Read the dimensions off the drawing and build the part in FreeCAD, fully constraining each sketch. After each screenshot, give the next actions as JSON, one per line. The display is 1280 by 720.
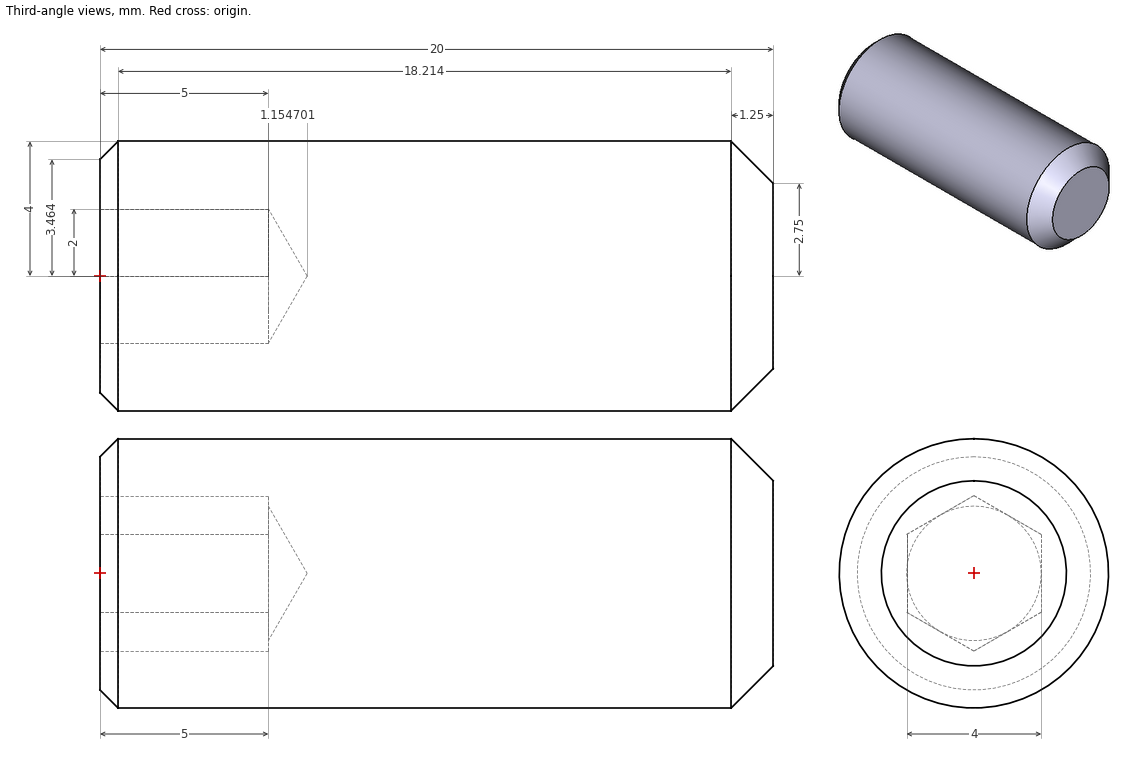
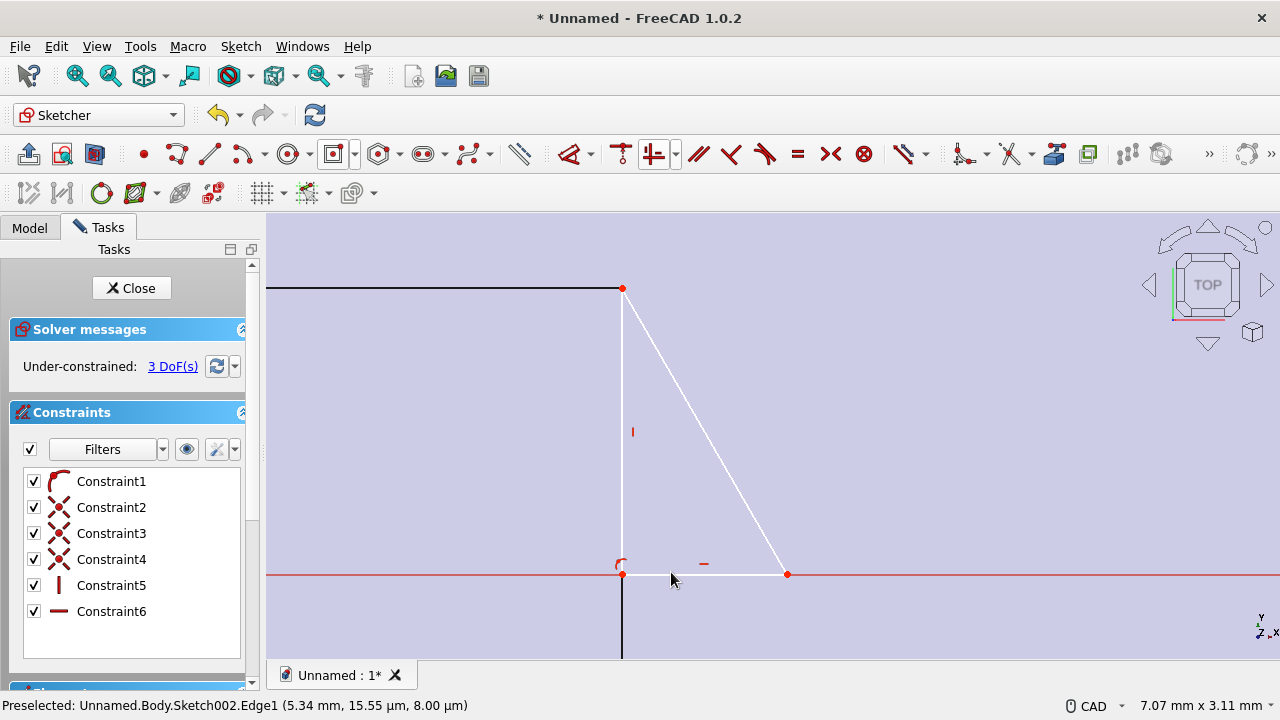
{"action": "left_click", "coordinate": [568, 154]}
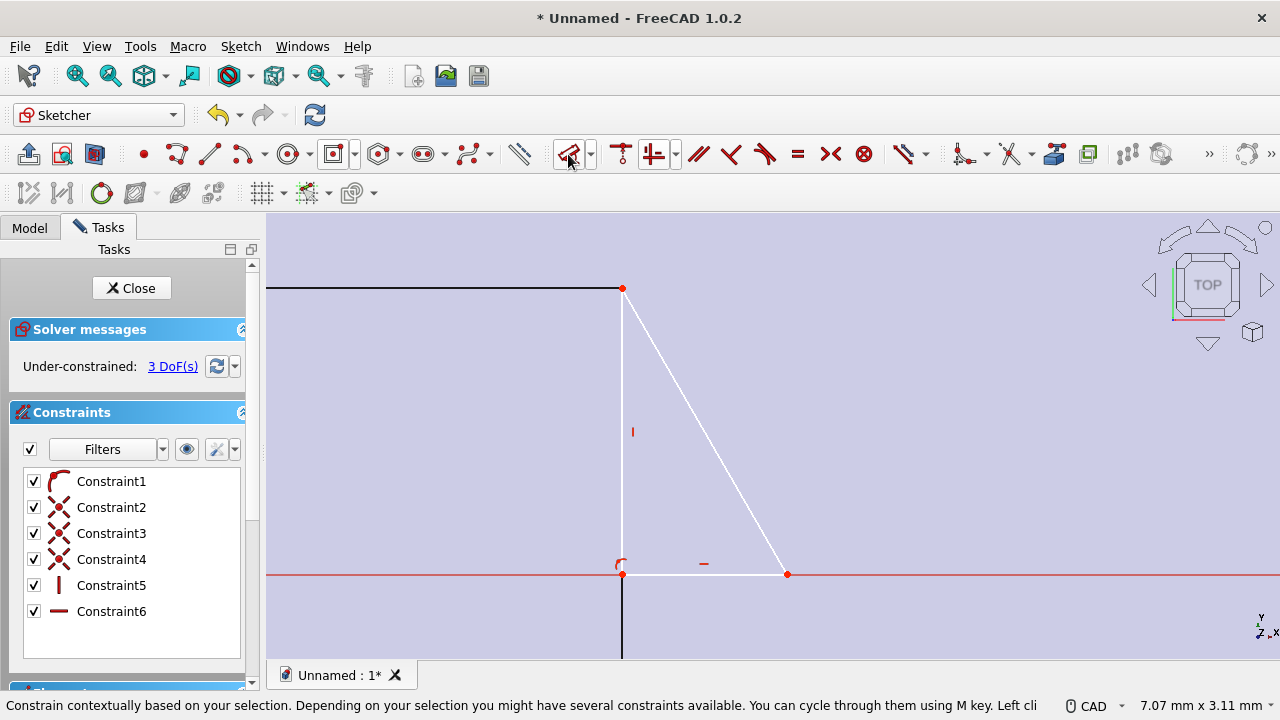
{"action": "left_click", "coordinate": [622, 375]}
{"action": "left_click", "coordinate": [588, 432]}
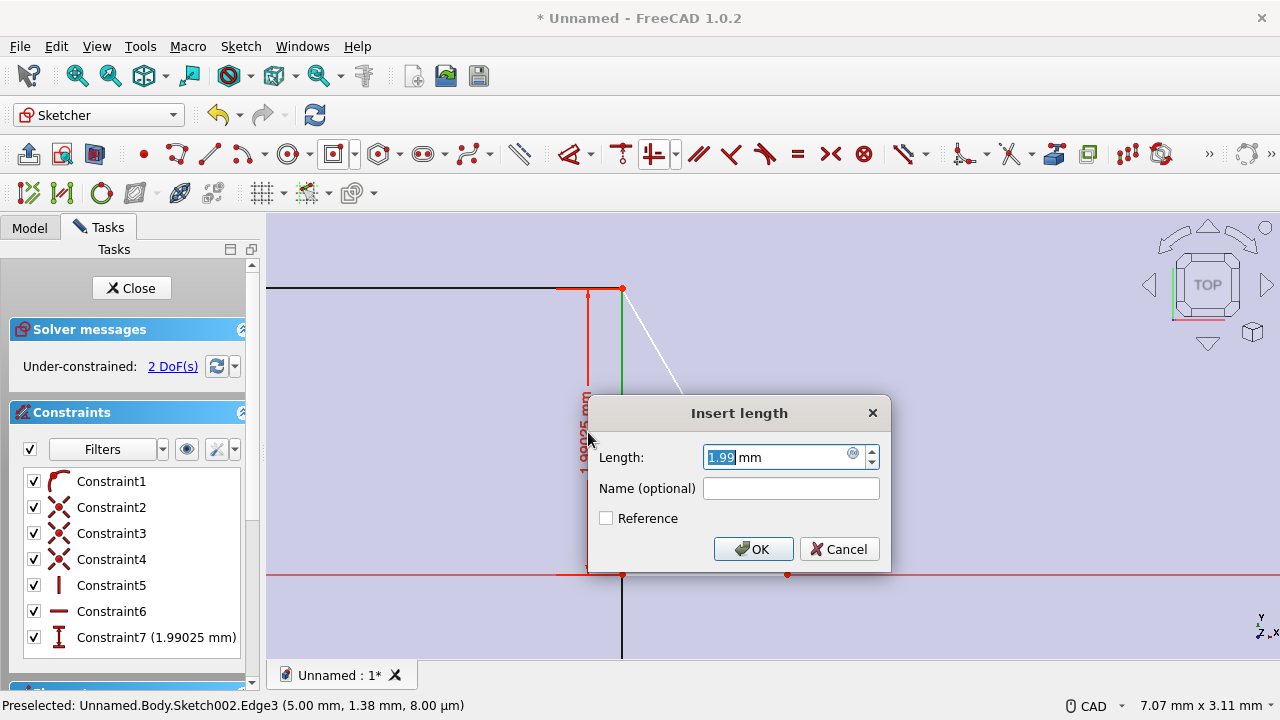
{"action": "type", "text": "2"}
{"action": "key", "text": "Return"}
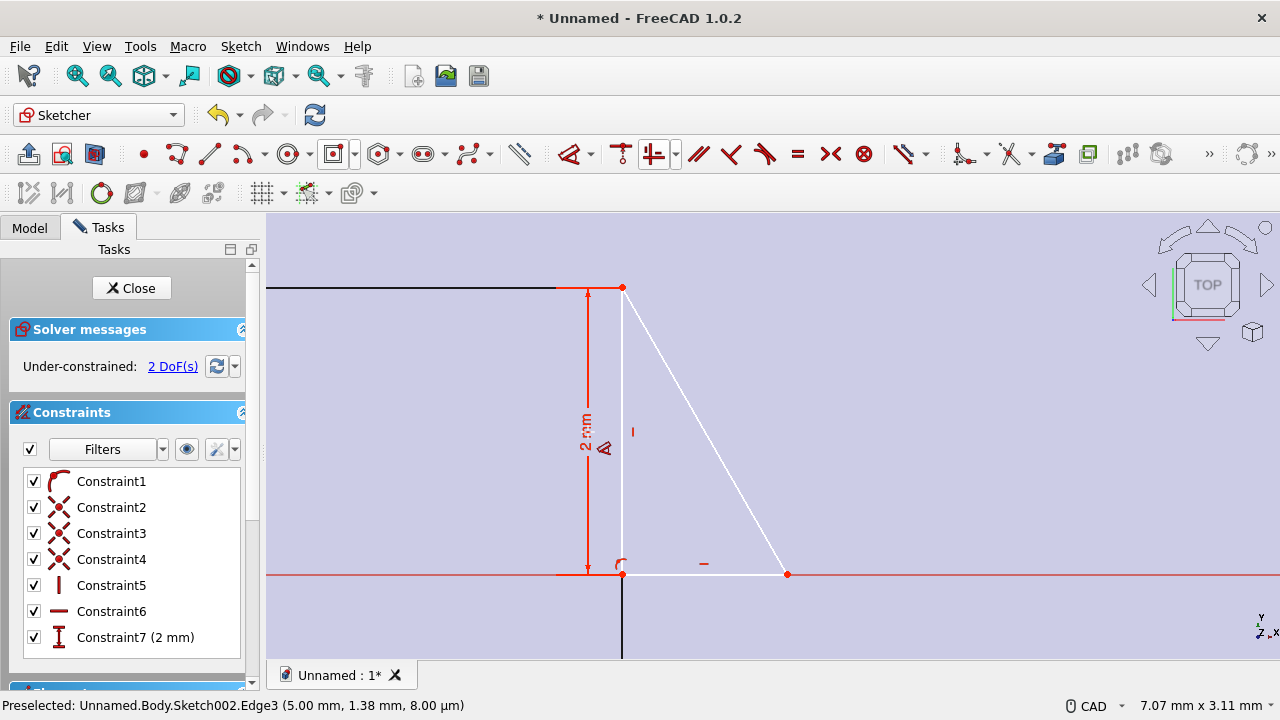
{"action": "left_click", "coordinate": [622, 575]}
{"action": "left_click", "coordinate": [458, 609]}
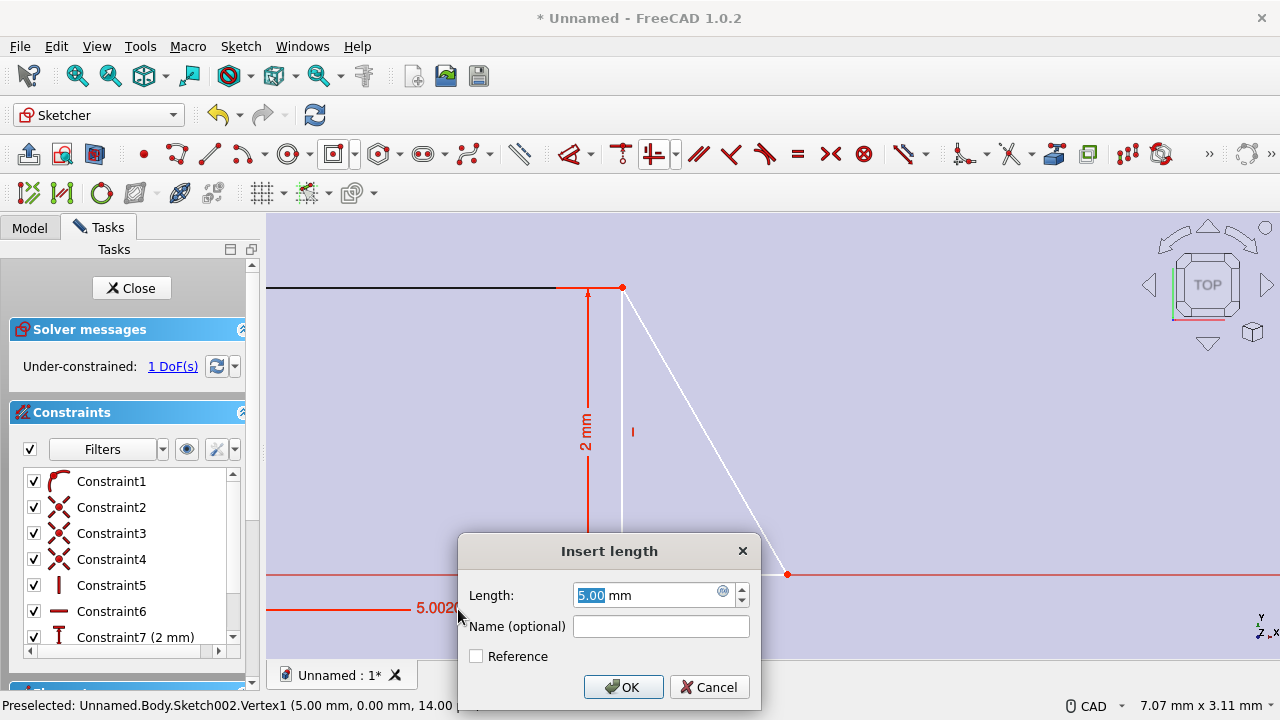
{"action": "type", "text": "5"}
{"action": "key", "text": "Return"}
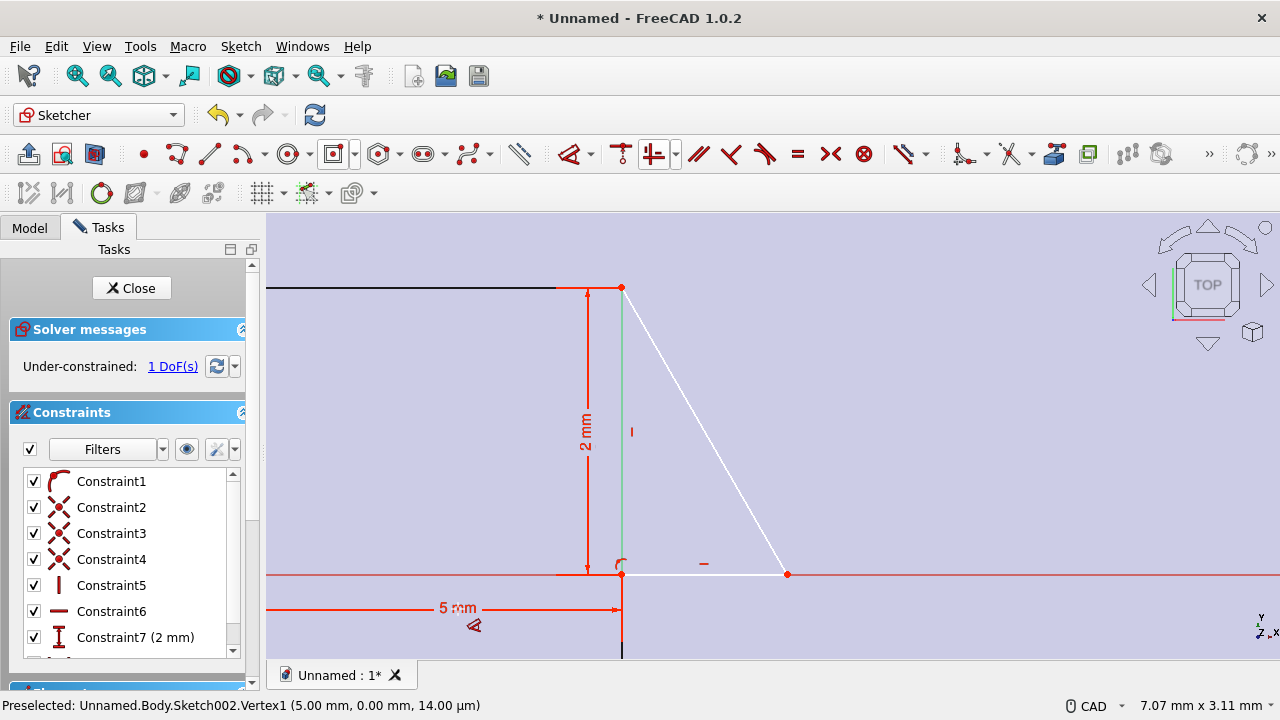
{"action": "left_click", "coordinate": [671, 575]}
{"action": "left_click", "coordinate": [704, 609]}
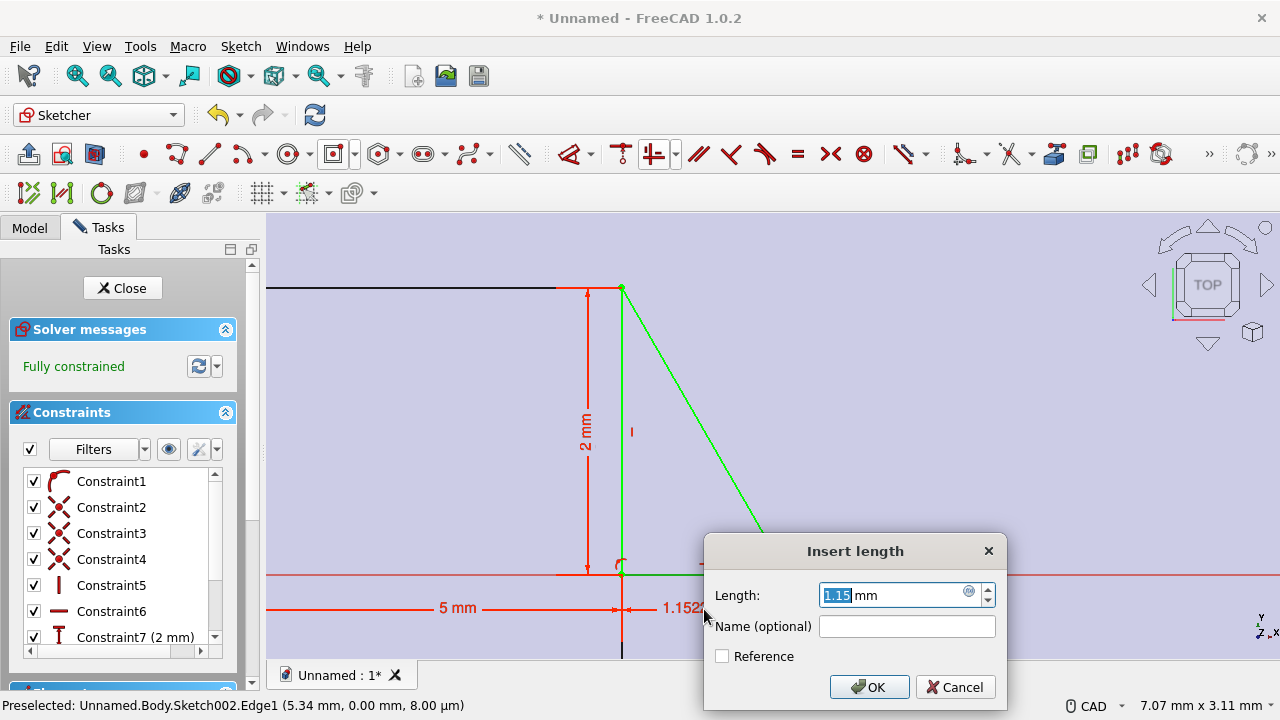
{"action": "type", "text": "1.154701"}
{"action": "key", "text": "Return"}
{"action": "key", "text": "Escape"}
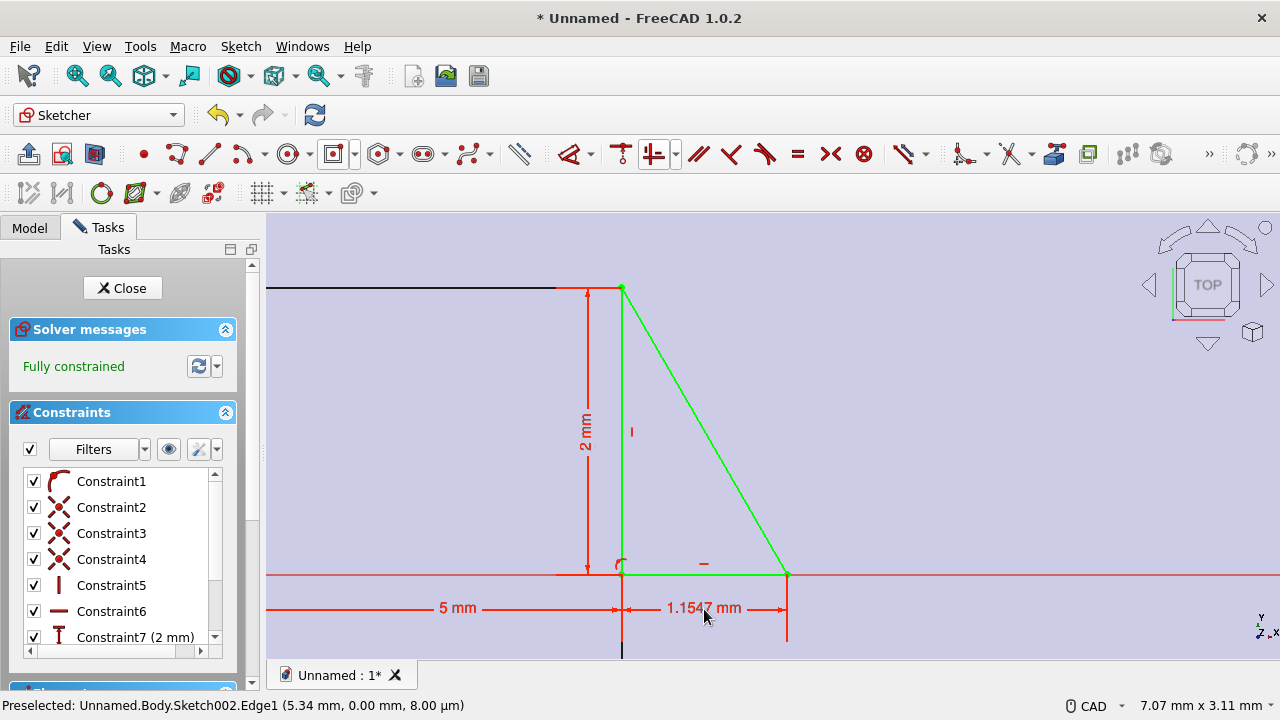
{"action": "left_click", "coordinate": [123, 288]}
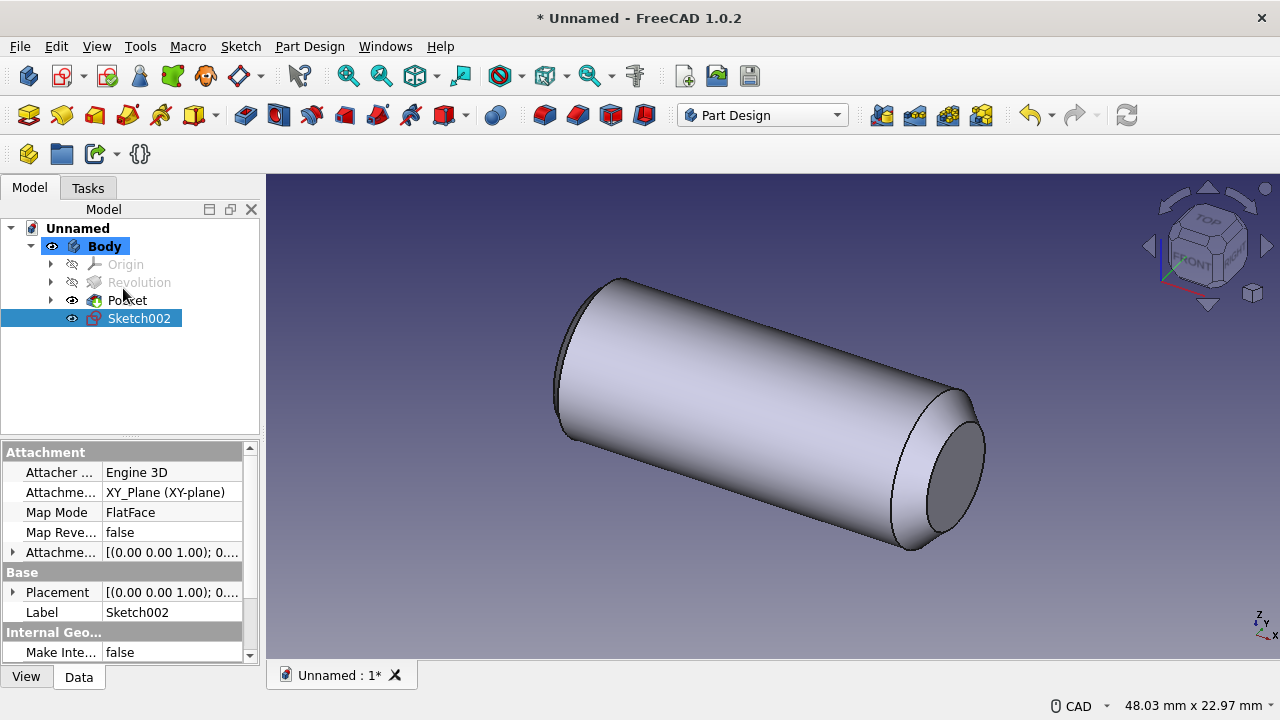
{"action": "left_click", "coordinate": [312, 116]}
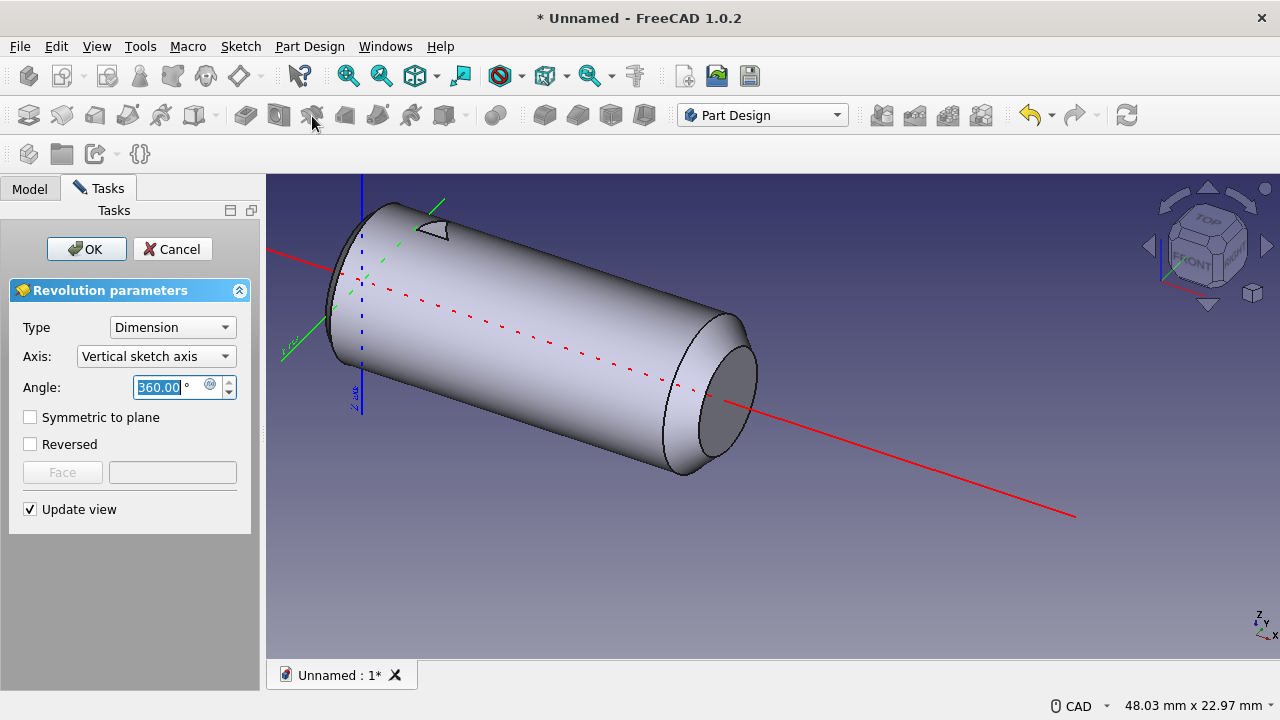
{"action": "left_click", "coordinate": [157, 356]}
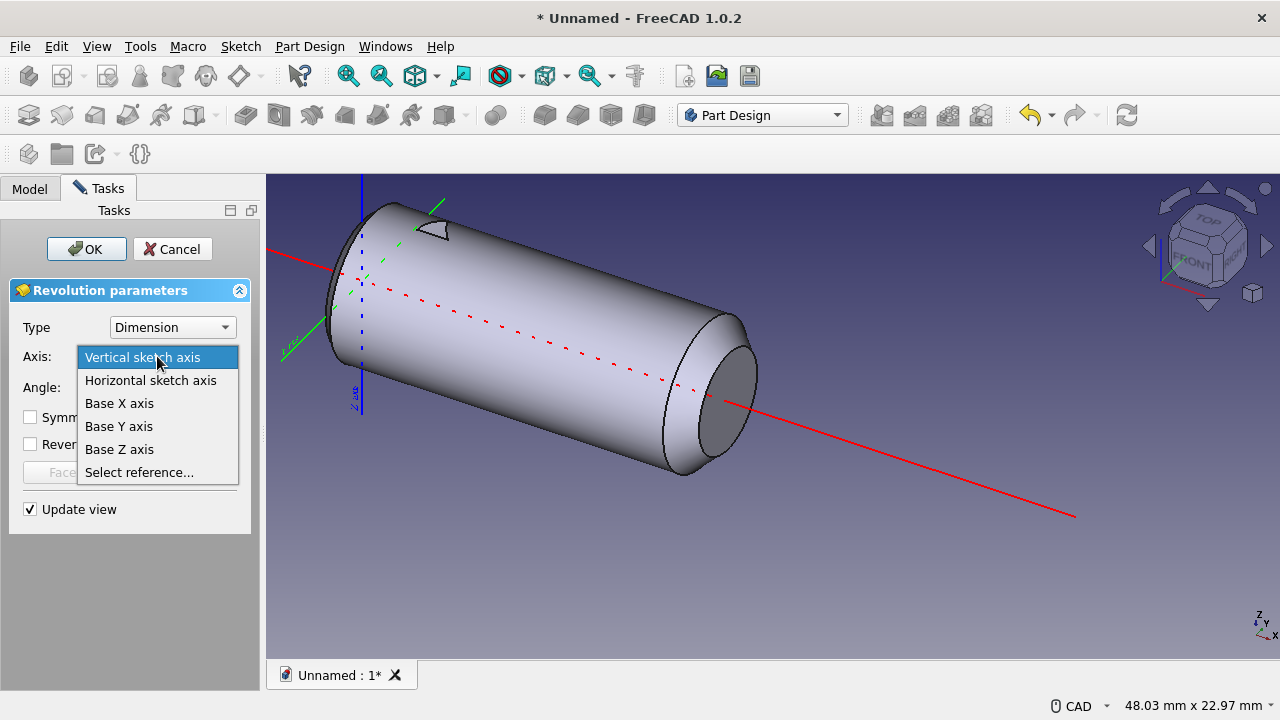
{"action": "left_click", "coordinate": [156, 380]}